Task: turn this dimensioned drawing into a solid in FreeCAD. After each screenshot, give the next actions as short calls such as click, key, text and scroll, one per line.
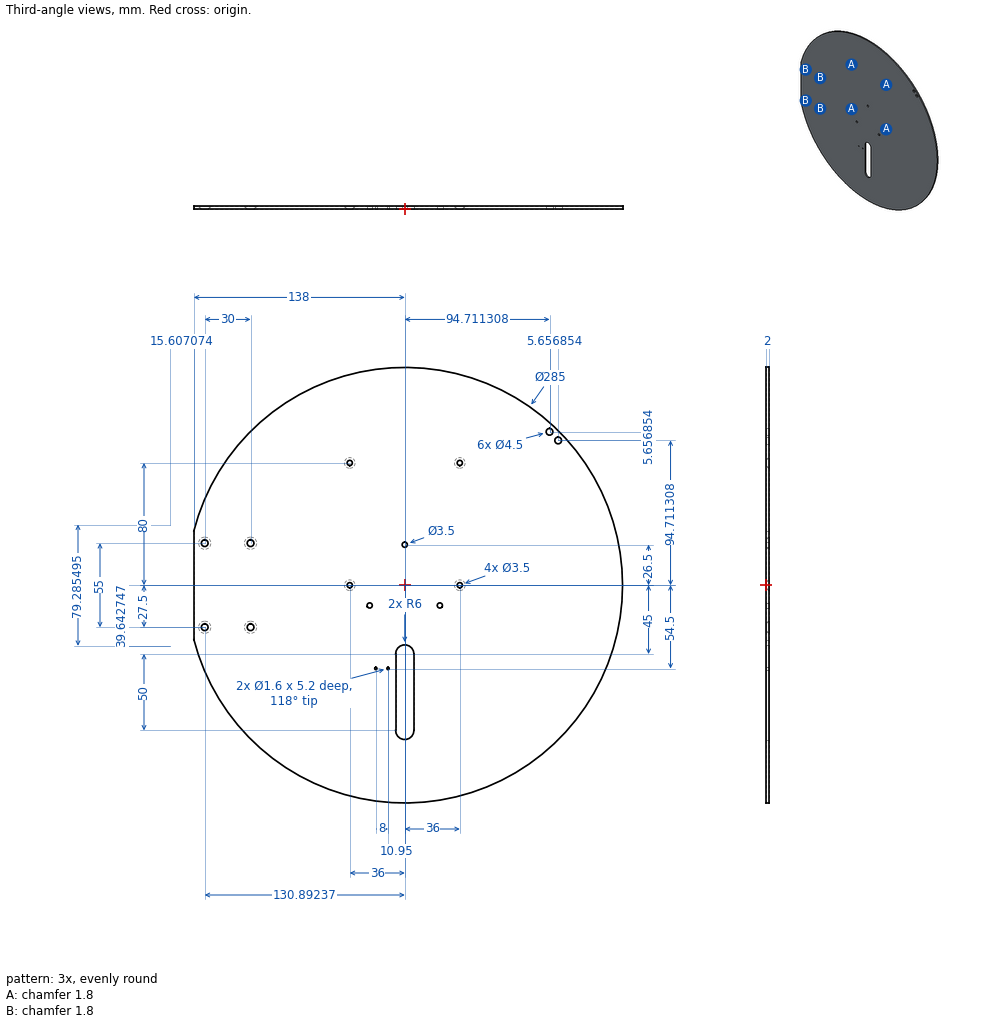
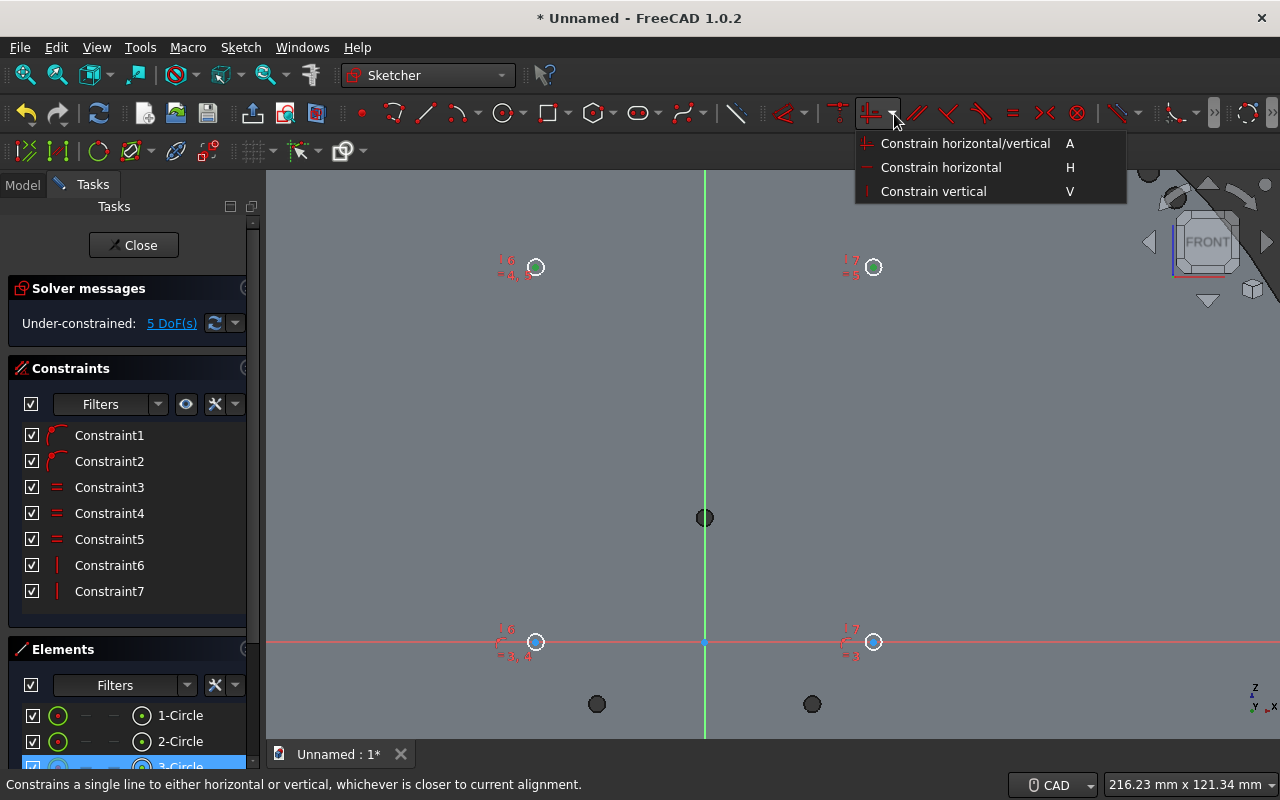
click(991, 167)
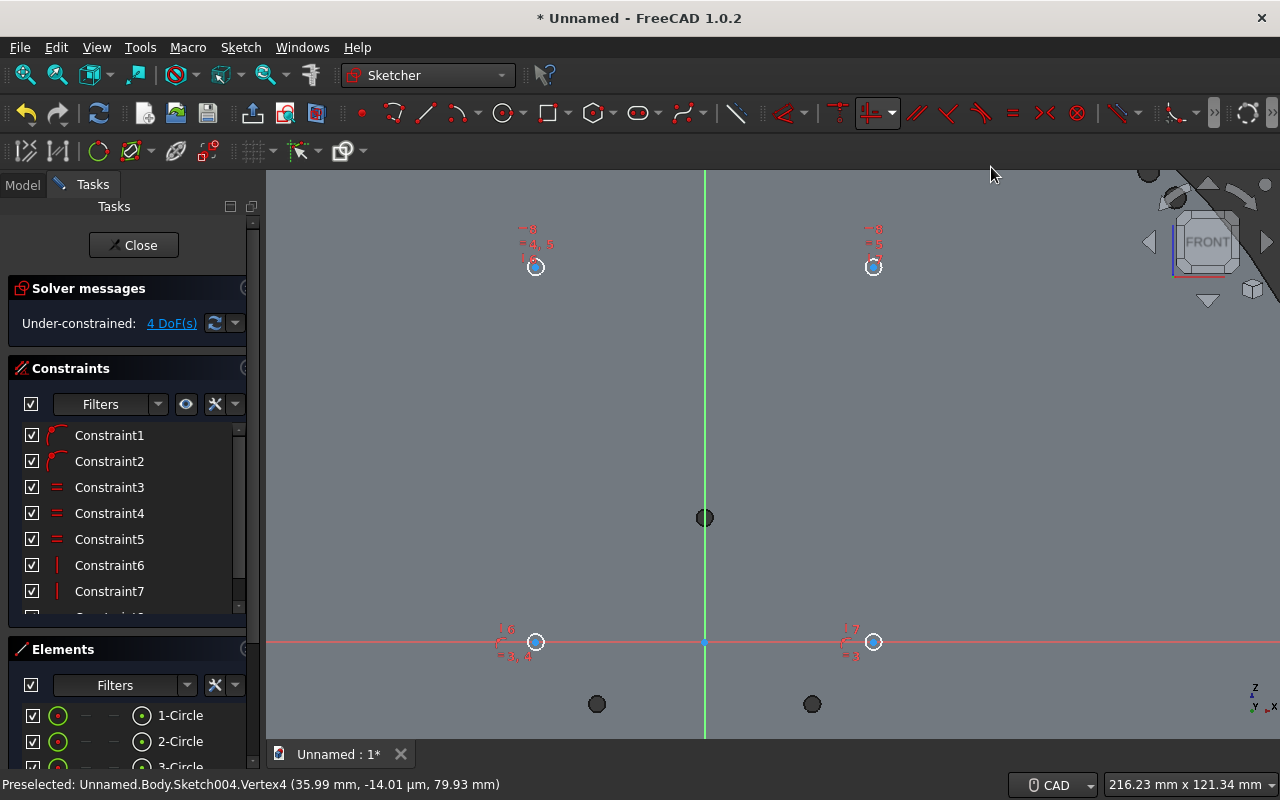
click(784, 114)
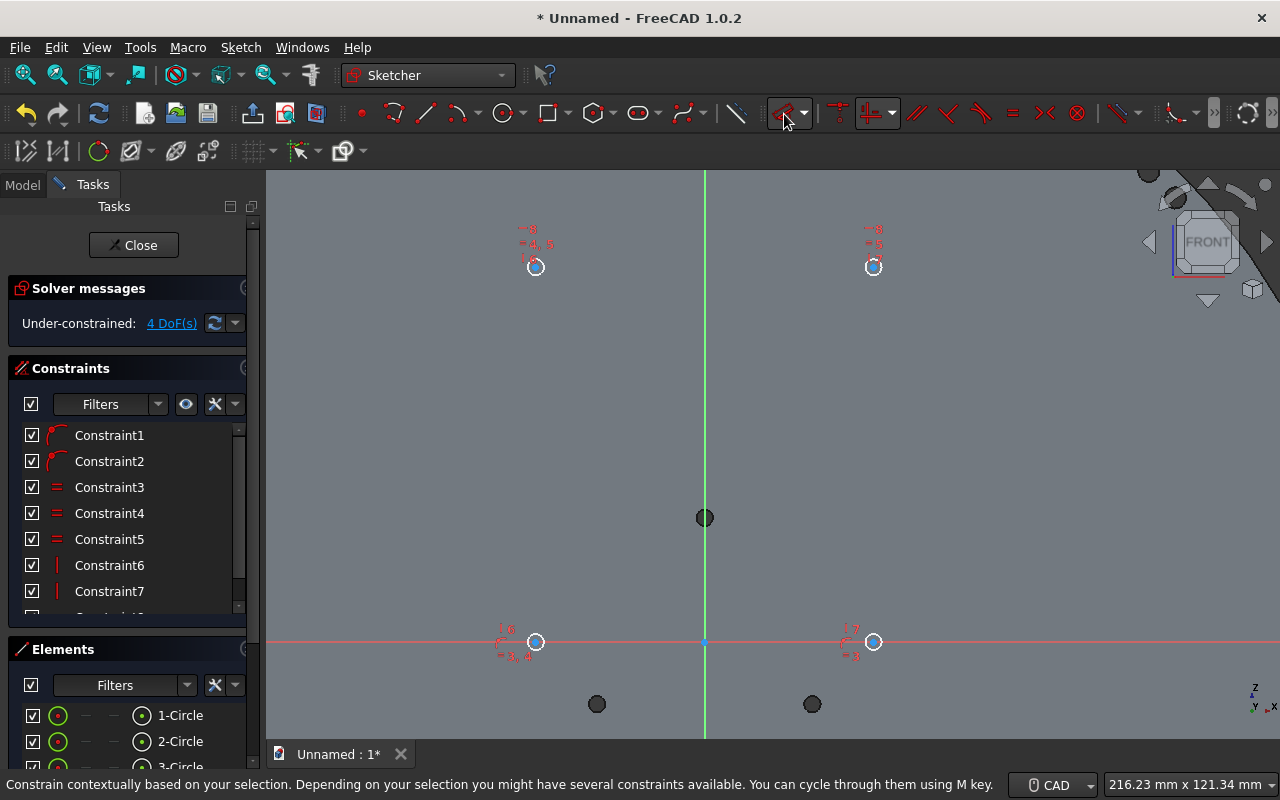
scroll(866, 642, up, 5)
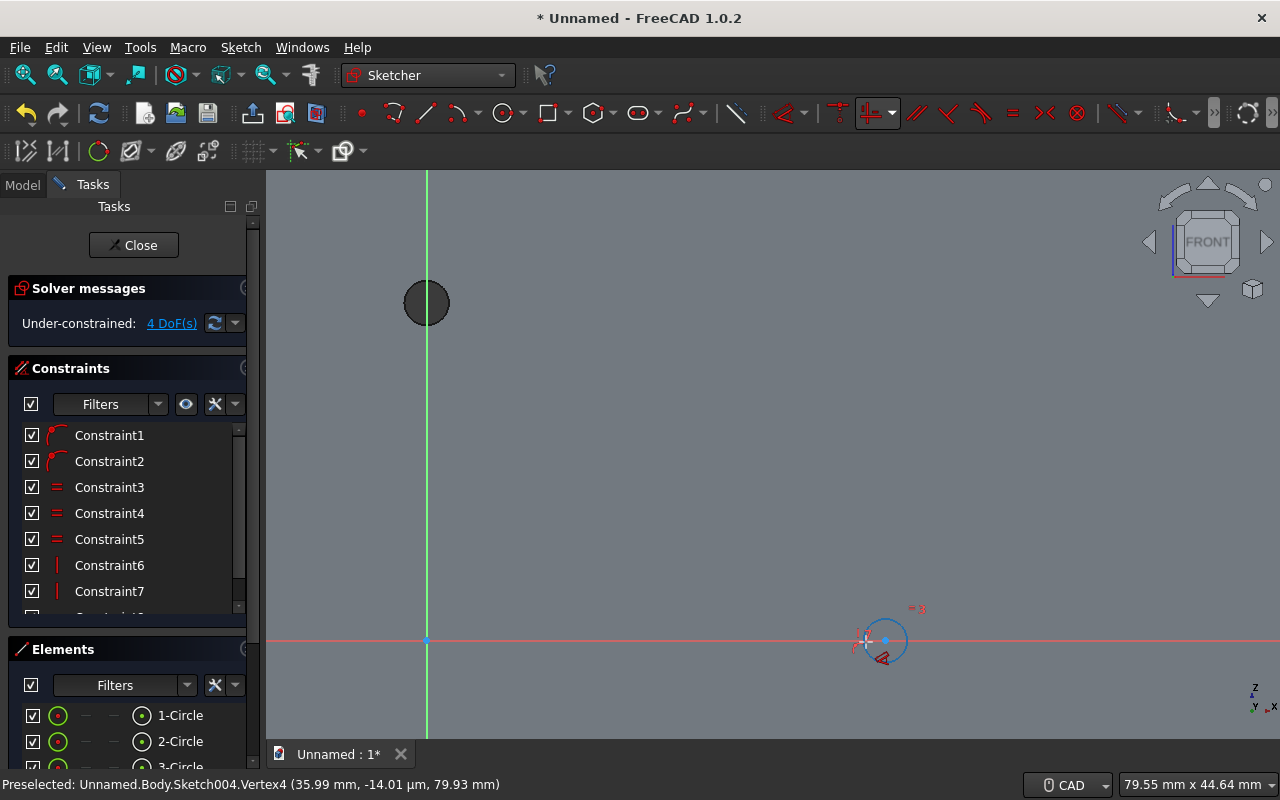
click(864, 640)
click(840, 613)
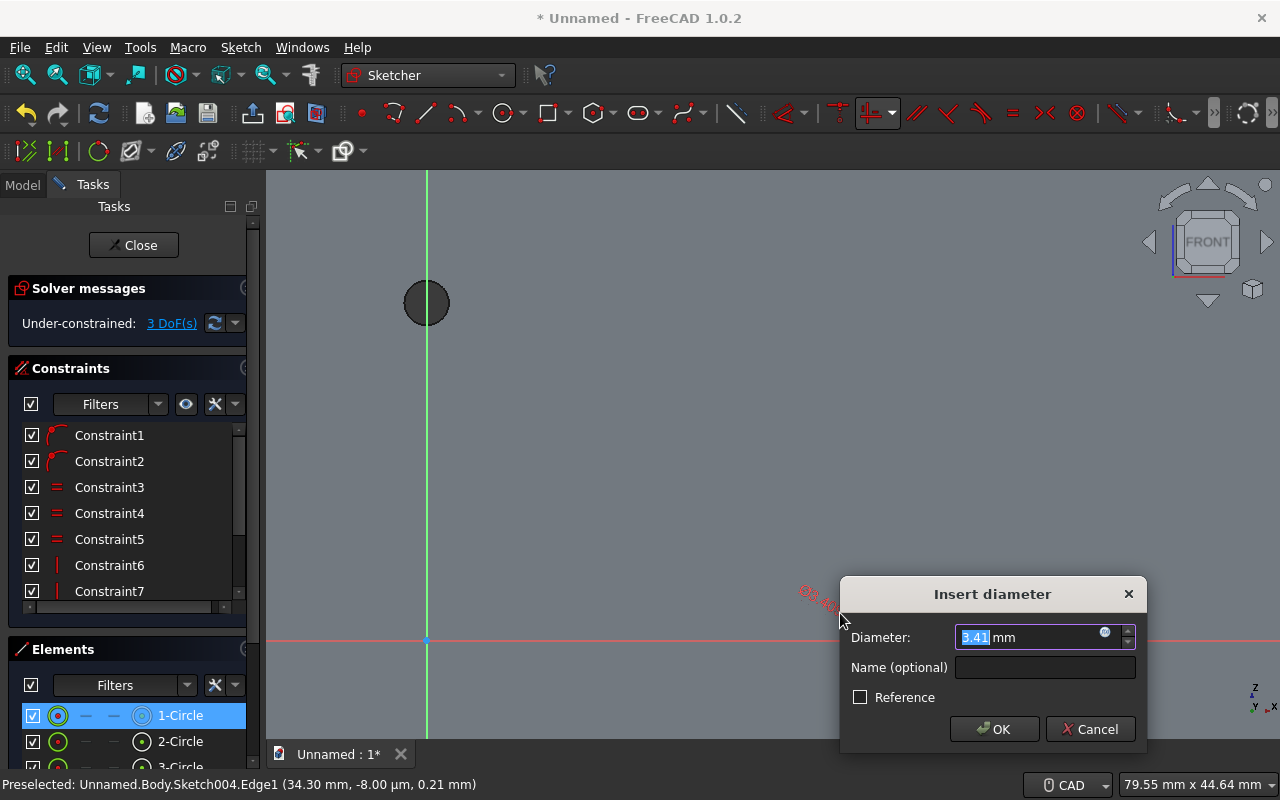
text(3.5)
key(Return)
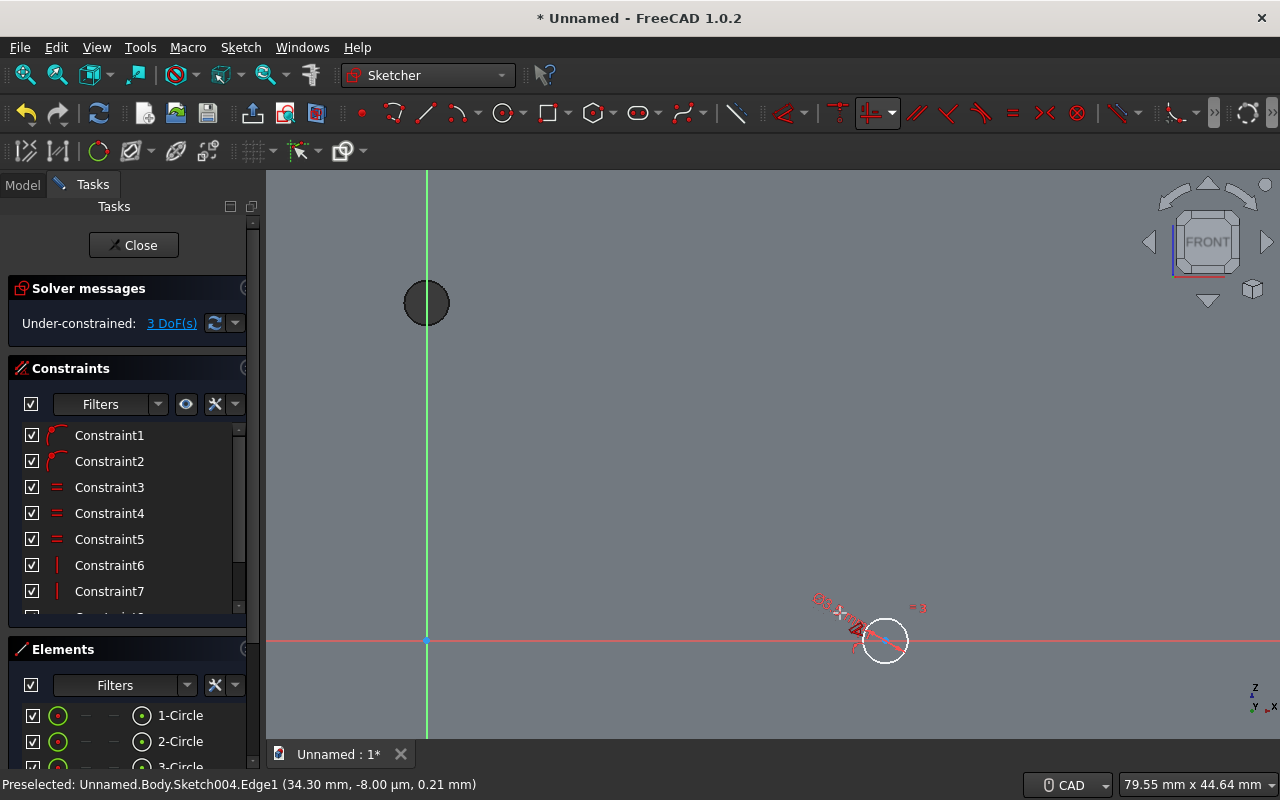
click(885, 641)
click(656, 675)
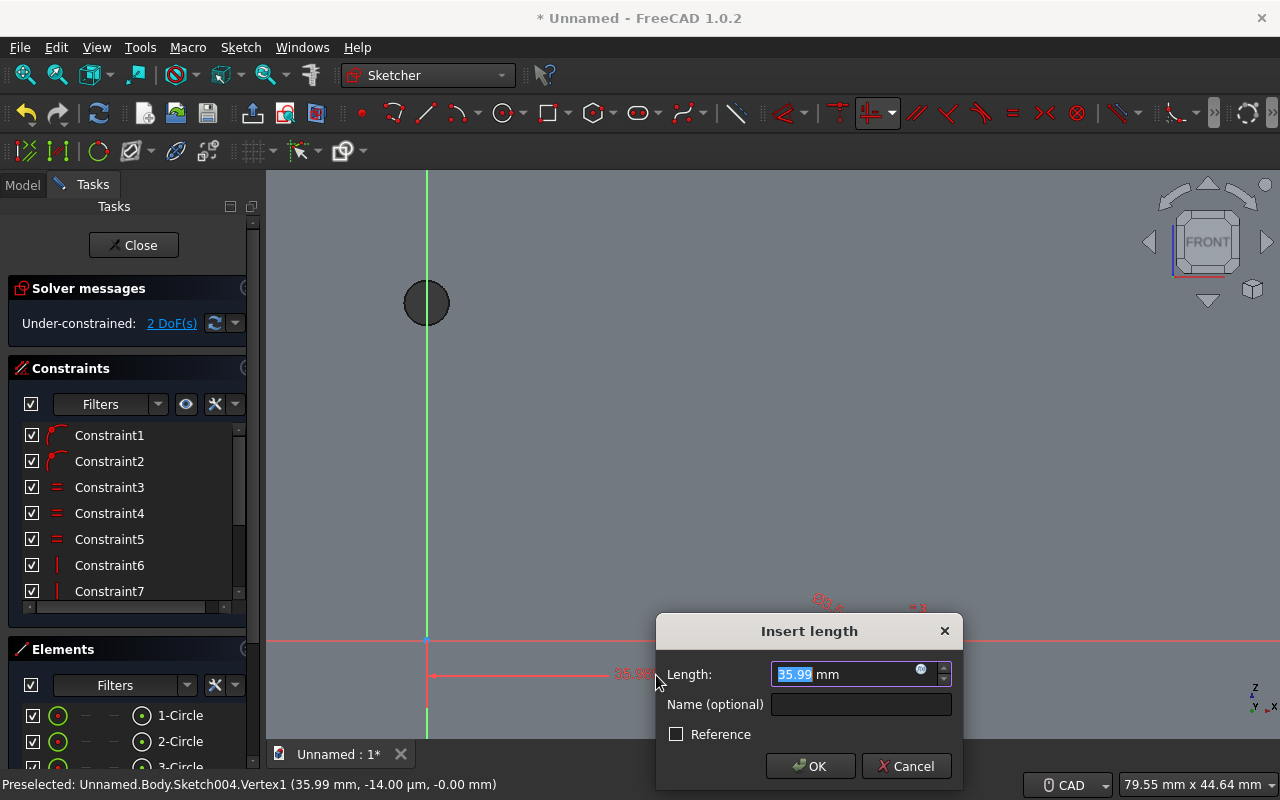
text(36)
key(Return)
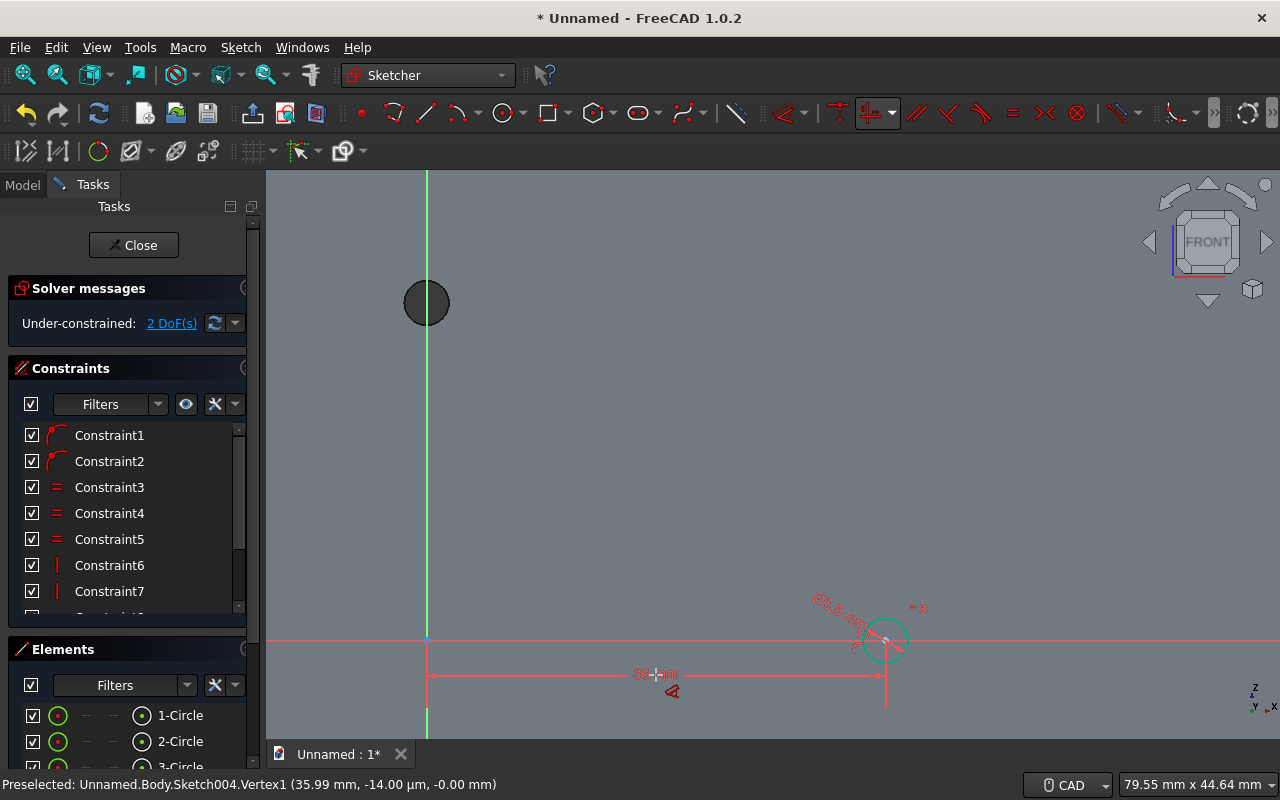
scroll(866, 643, down, 5)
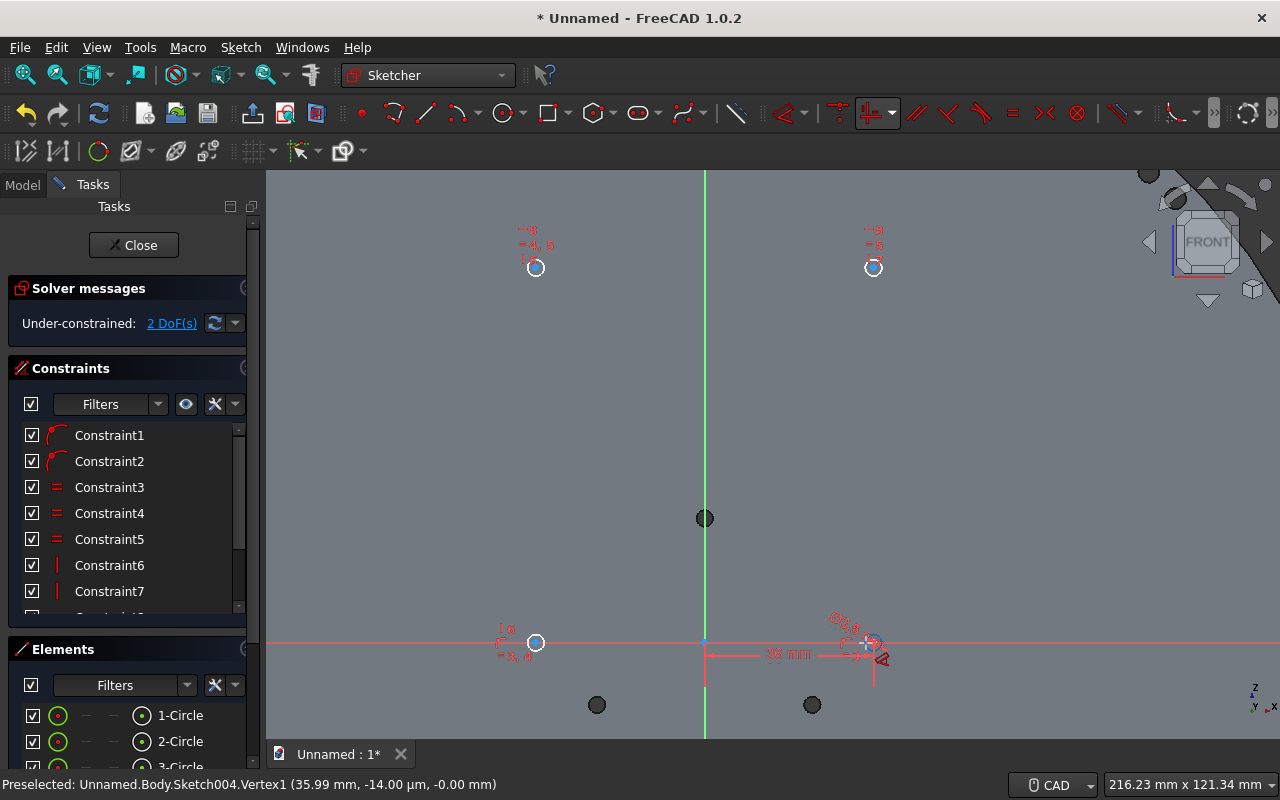
click(536, 643)
click(620, 677)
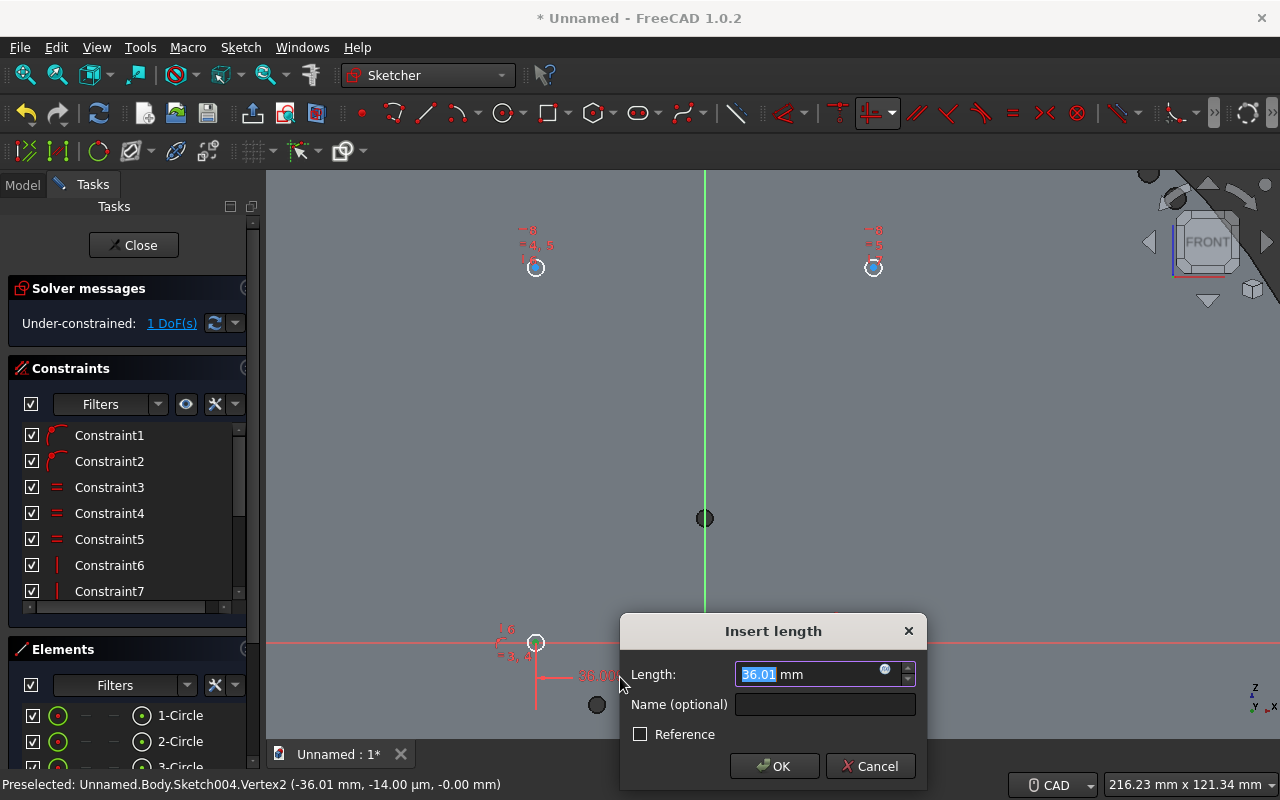
text(36)
key(Return)